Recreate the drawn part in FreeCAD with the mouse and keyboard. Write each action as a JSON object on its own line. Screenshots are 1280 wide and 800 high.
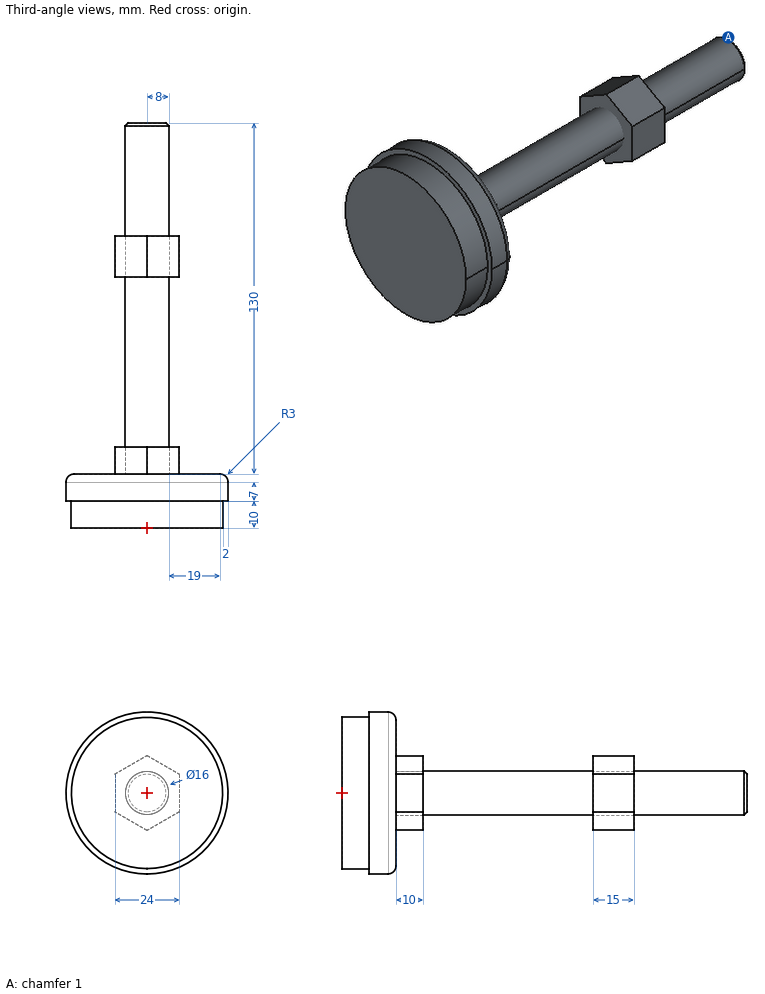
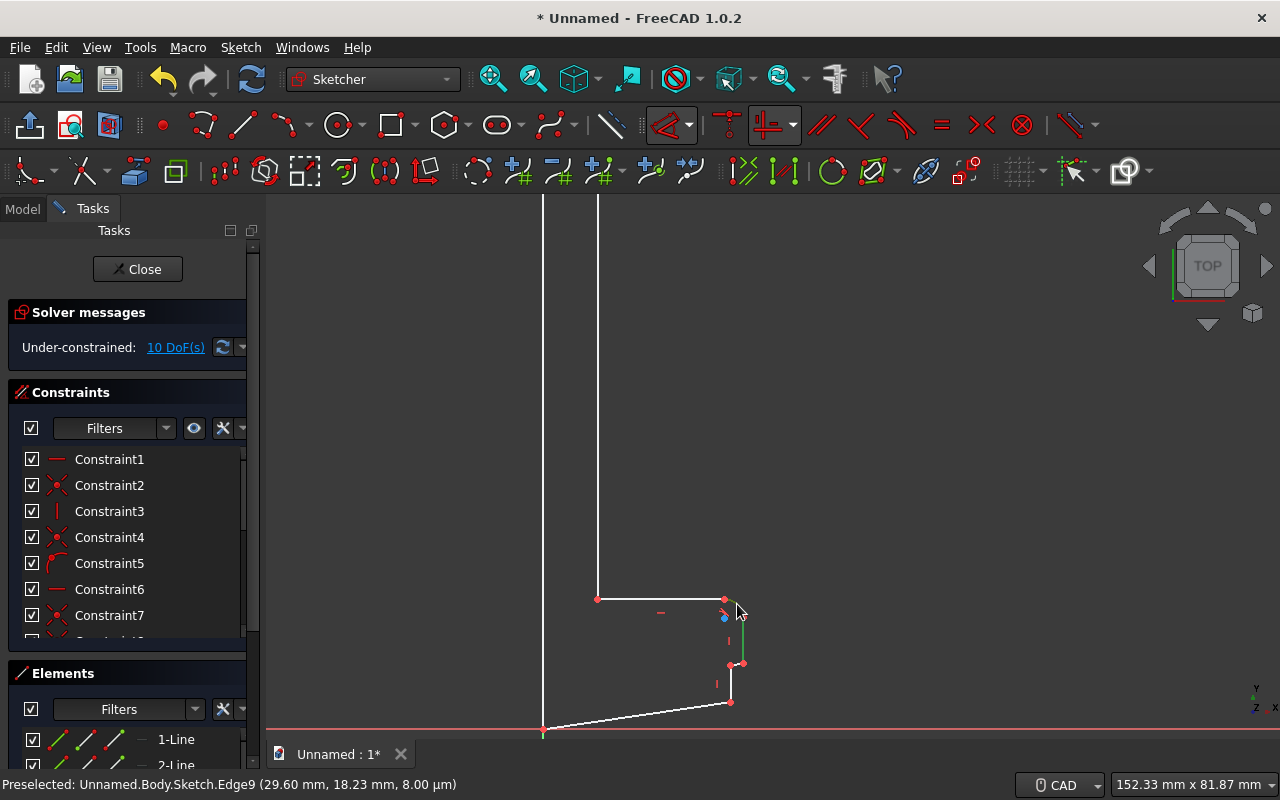
{"action": "left_click", "coordinate": [902, 126]}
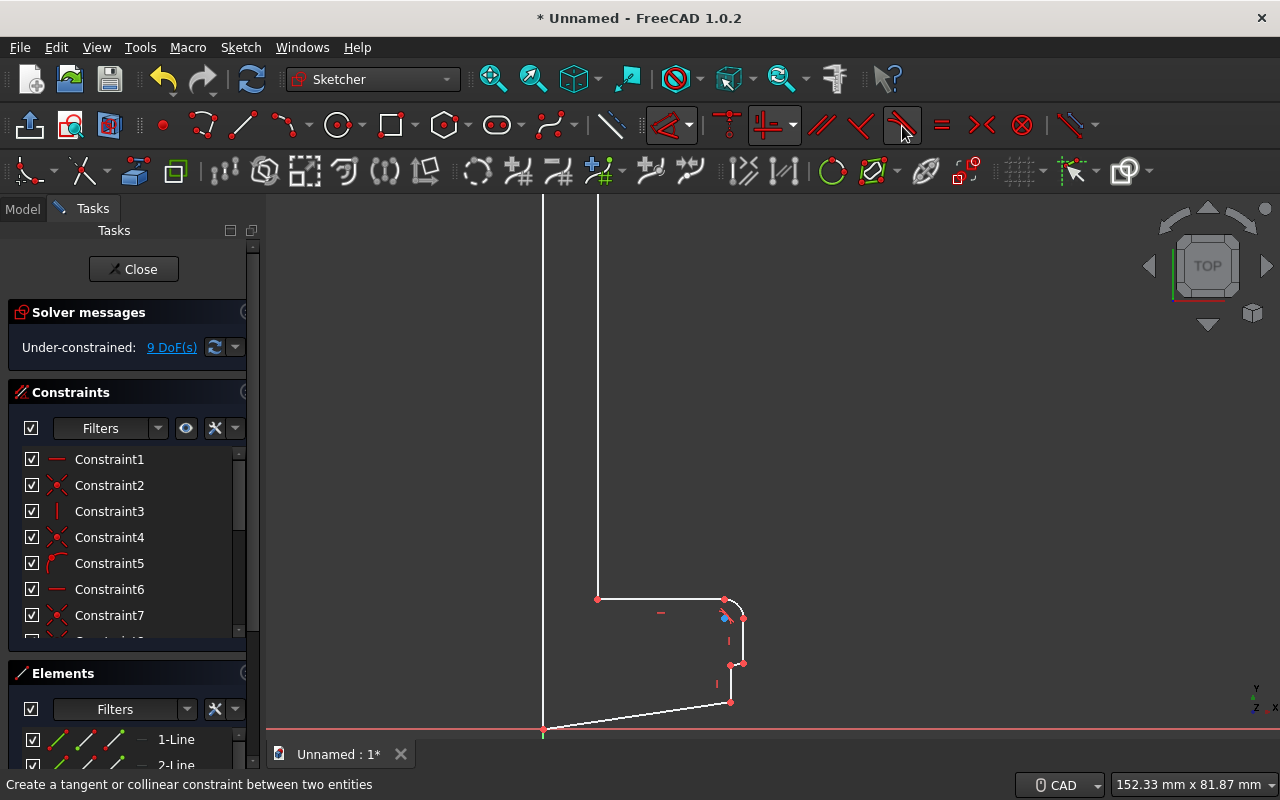
{"action": "left_click", "coordinate": [675, 710]}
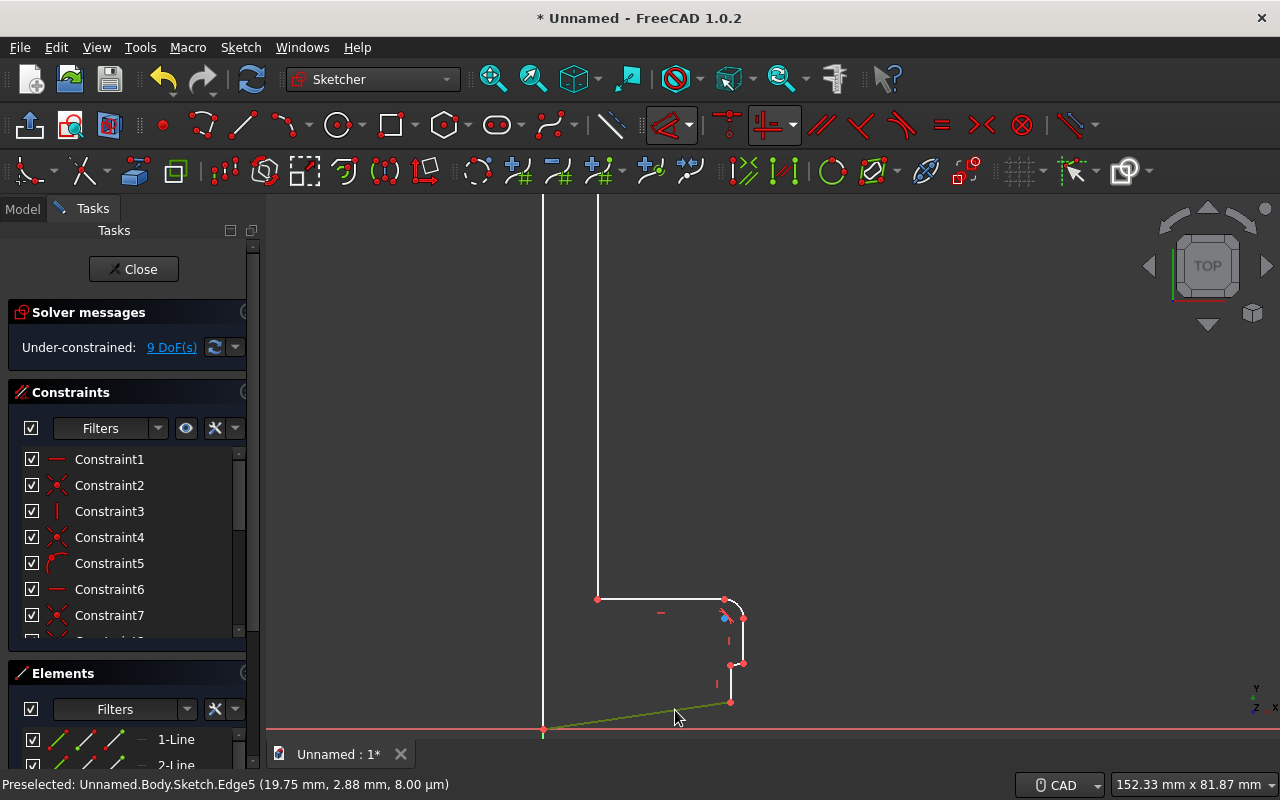
{"action": "key", "text": "h"}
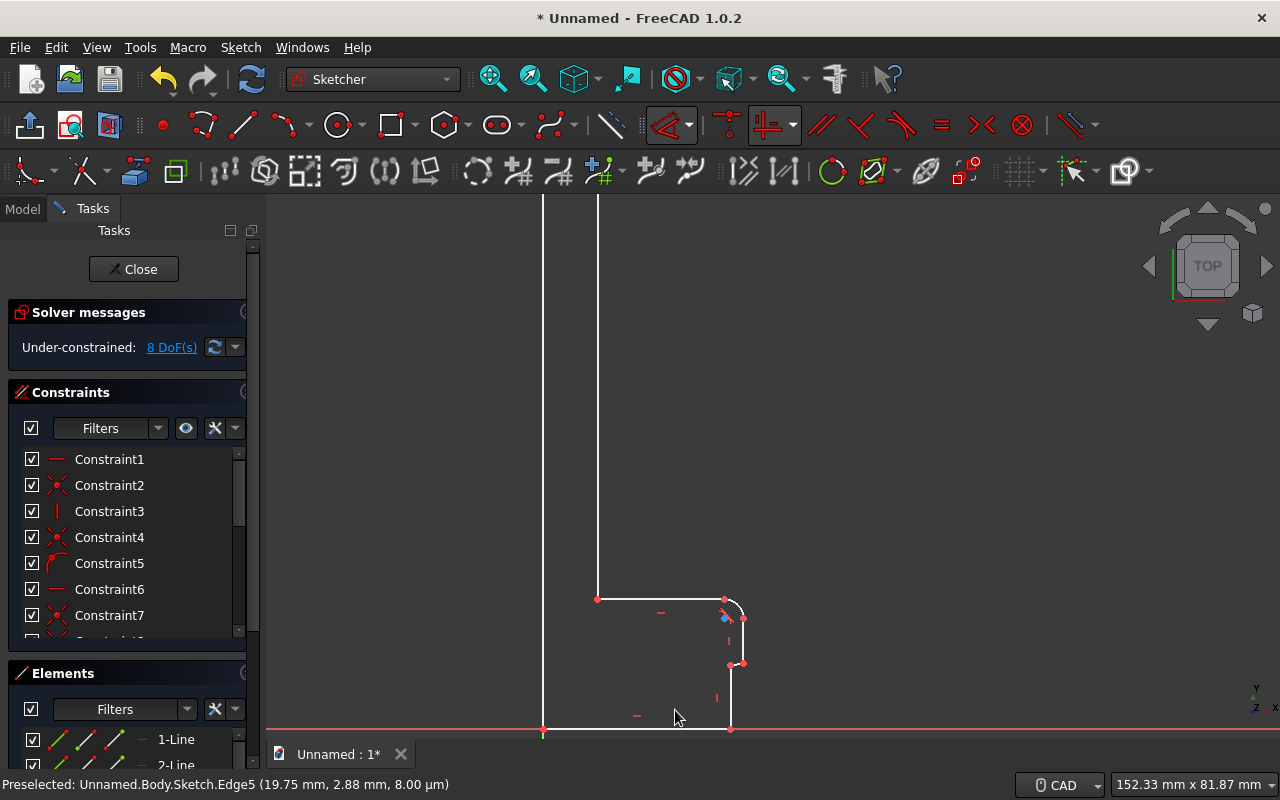
{"action": "scroll", "coordinate": [737, 664], "scroll_direction": "up", "scroll_amount": 4}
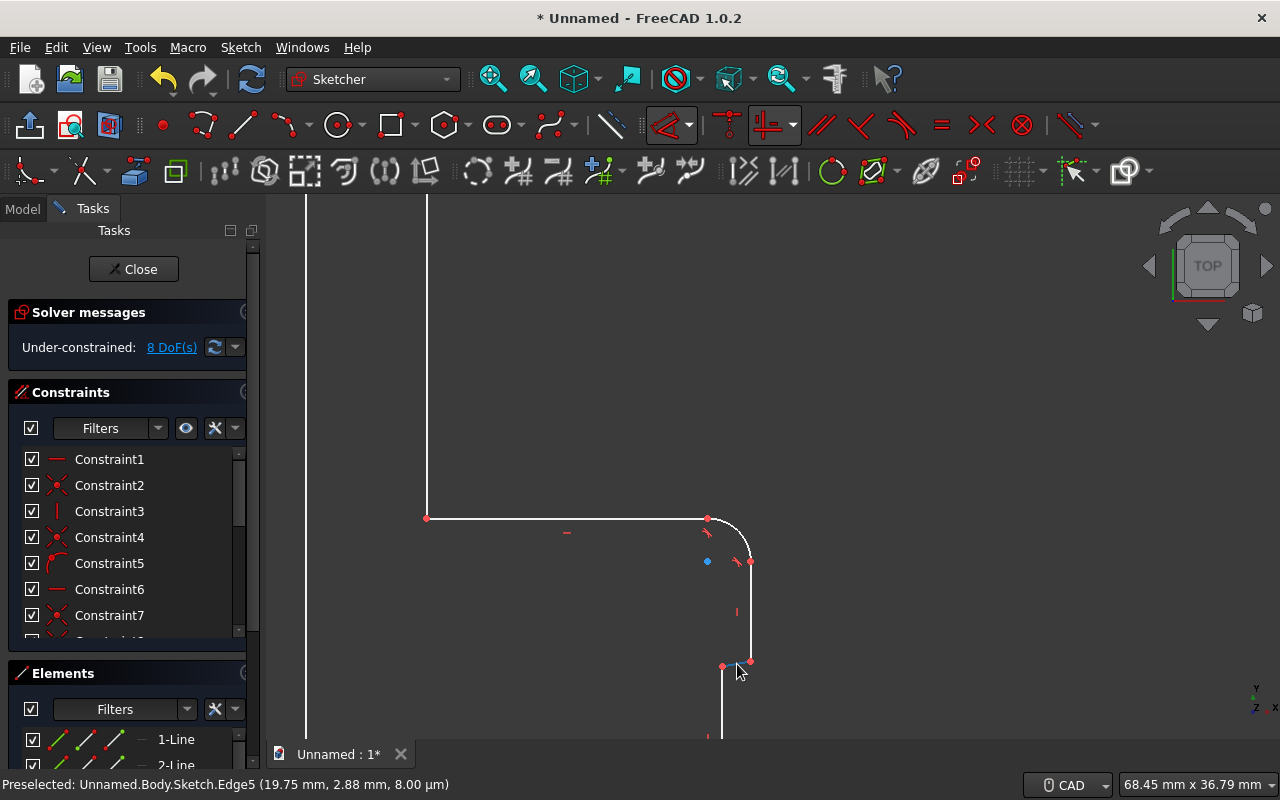
{"action": "left_click", "coordinate": [737, 664]}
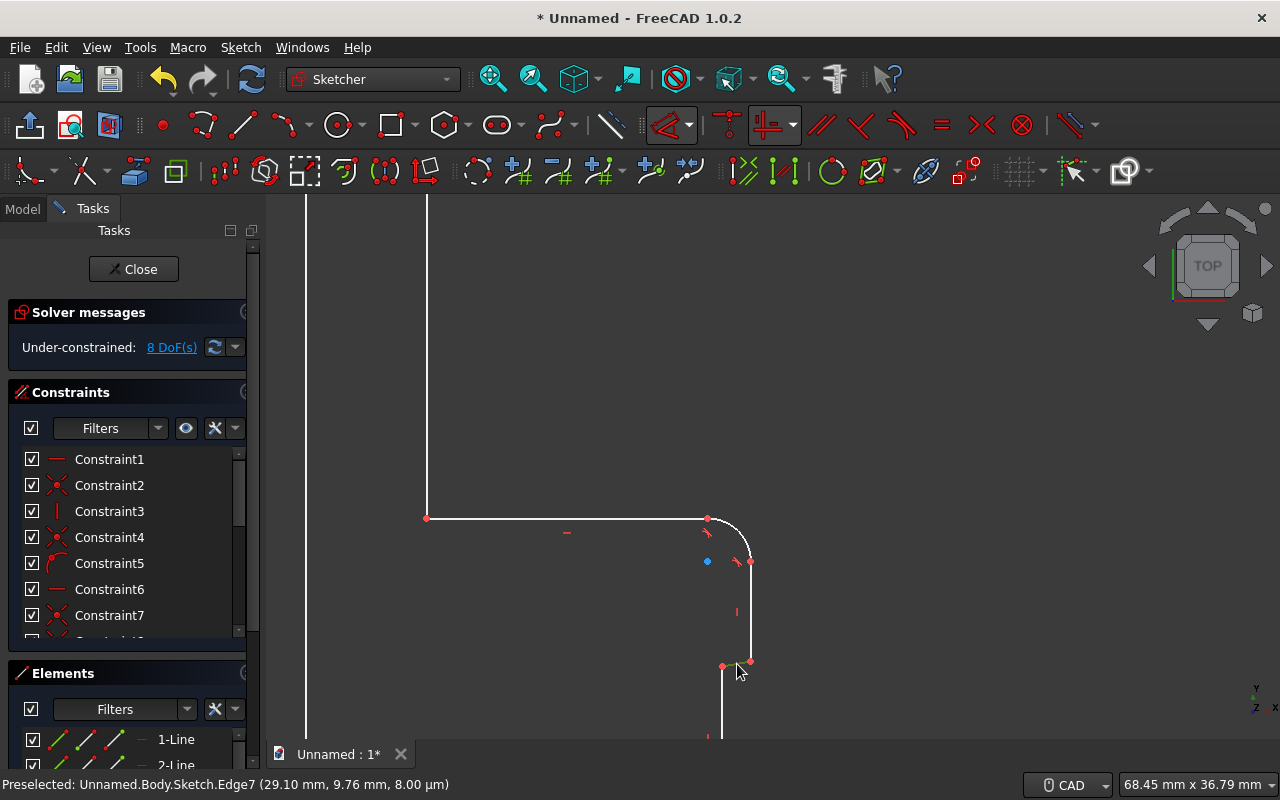
{"action": "left_click", "coordinate": [796, 126]}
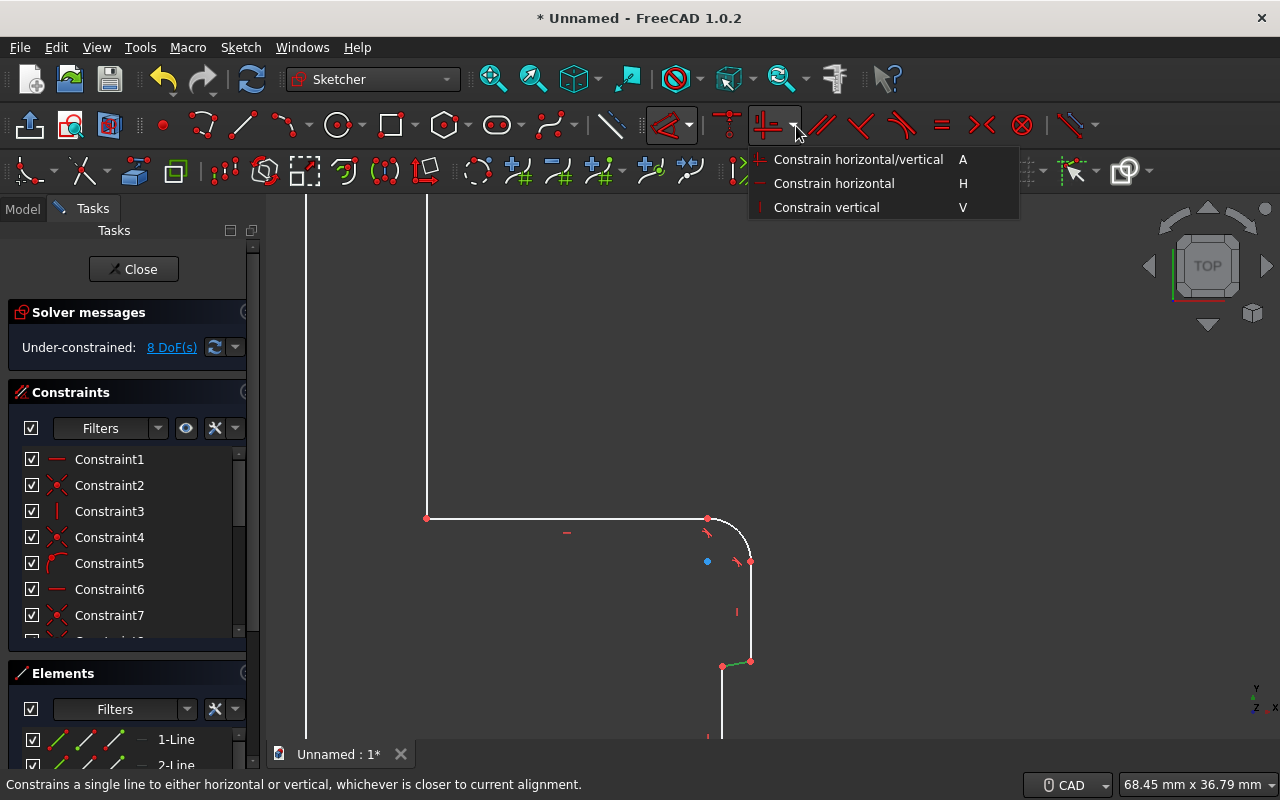
{"action": "left_click", "coordinate": [884, 183]}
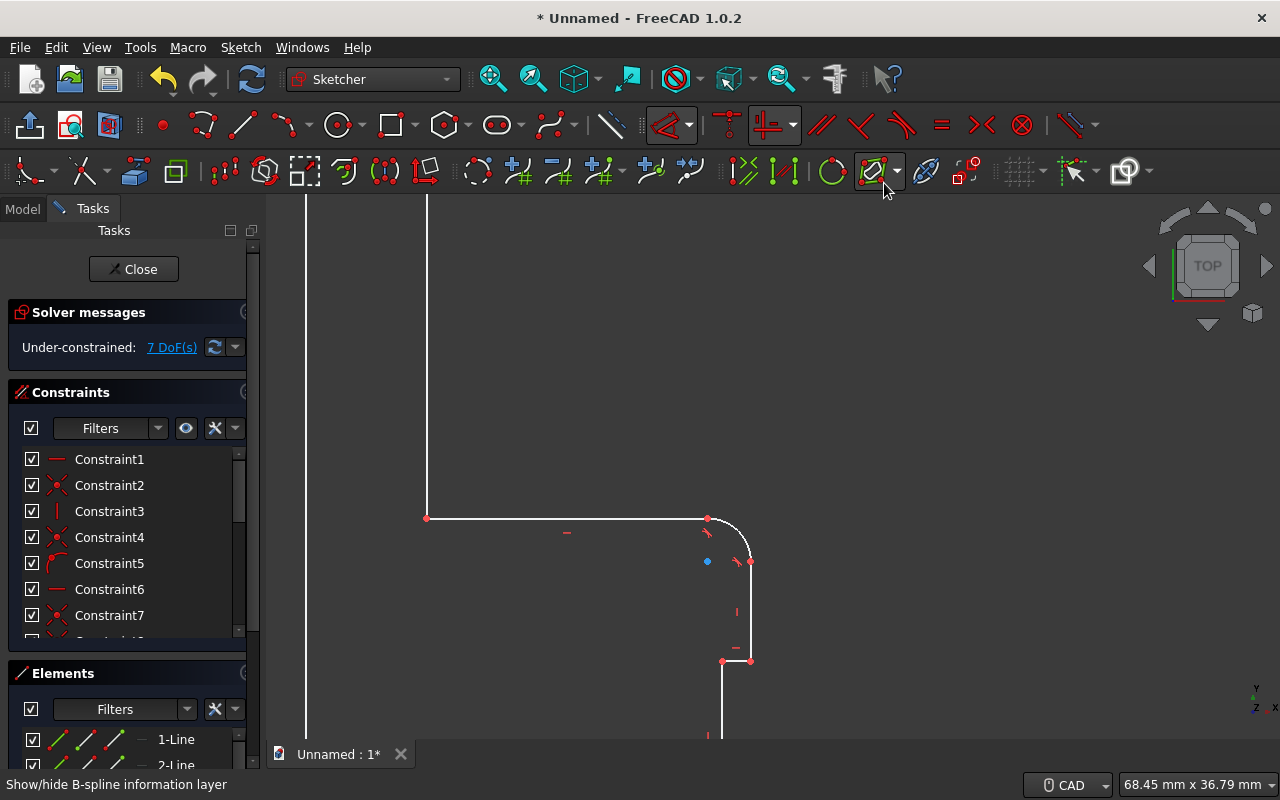
{"action": "left_click", "coordinate": [746, 542]}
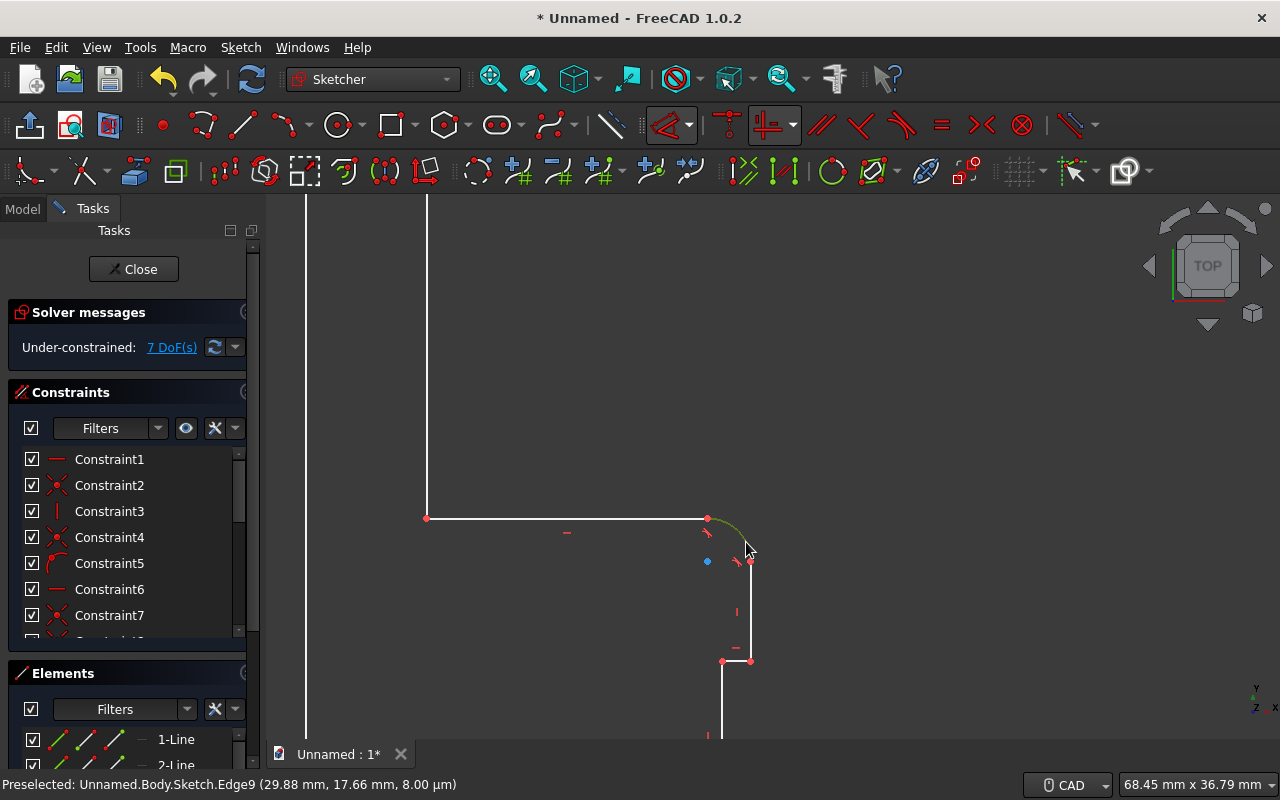
{"action": "key", "text": "k r"}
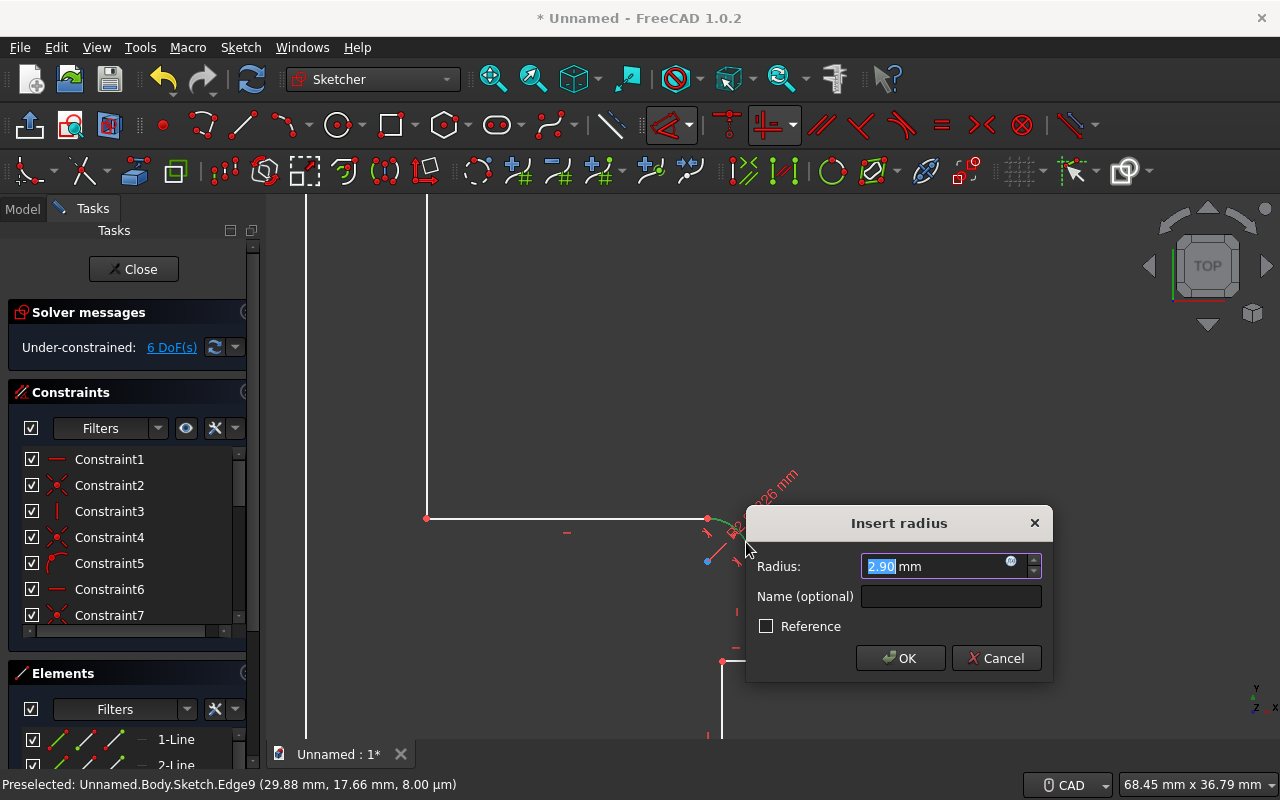
{"action": "type", "text": "3"}
{"action": "key", "text": "Return"}